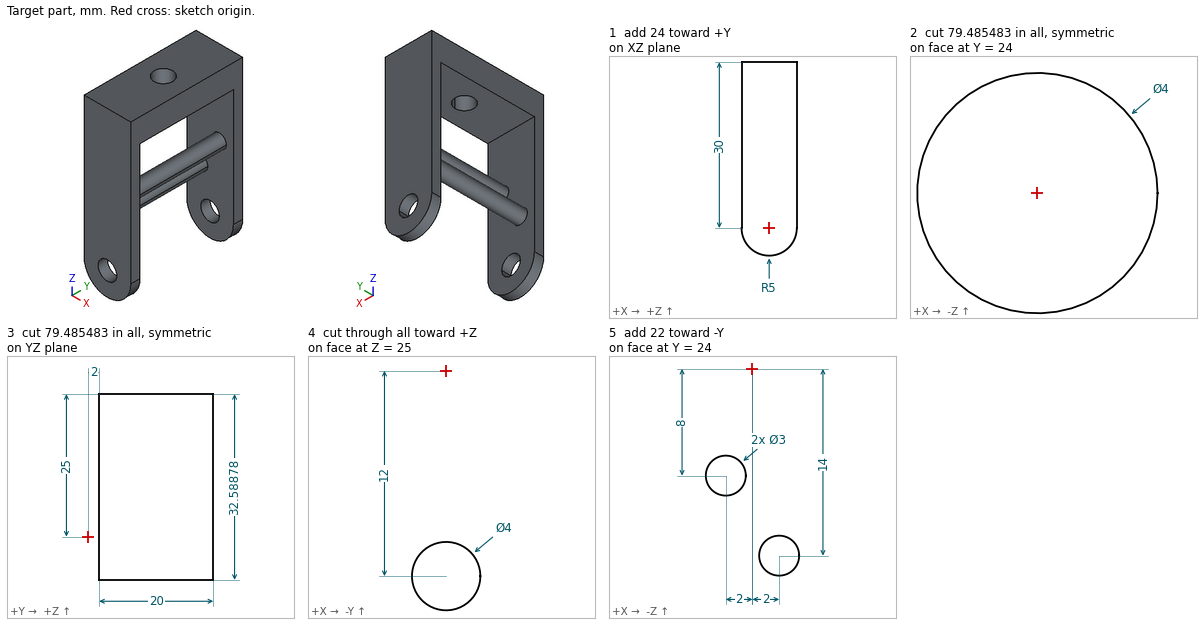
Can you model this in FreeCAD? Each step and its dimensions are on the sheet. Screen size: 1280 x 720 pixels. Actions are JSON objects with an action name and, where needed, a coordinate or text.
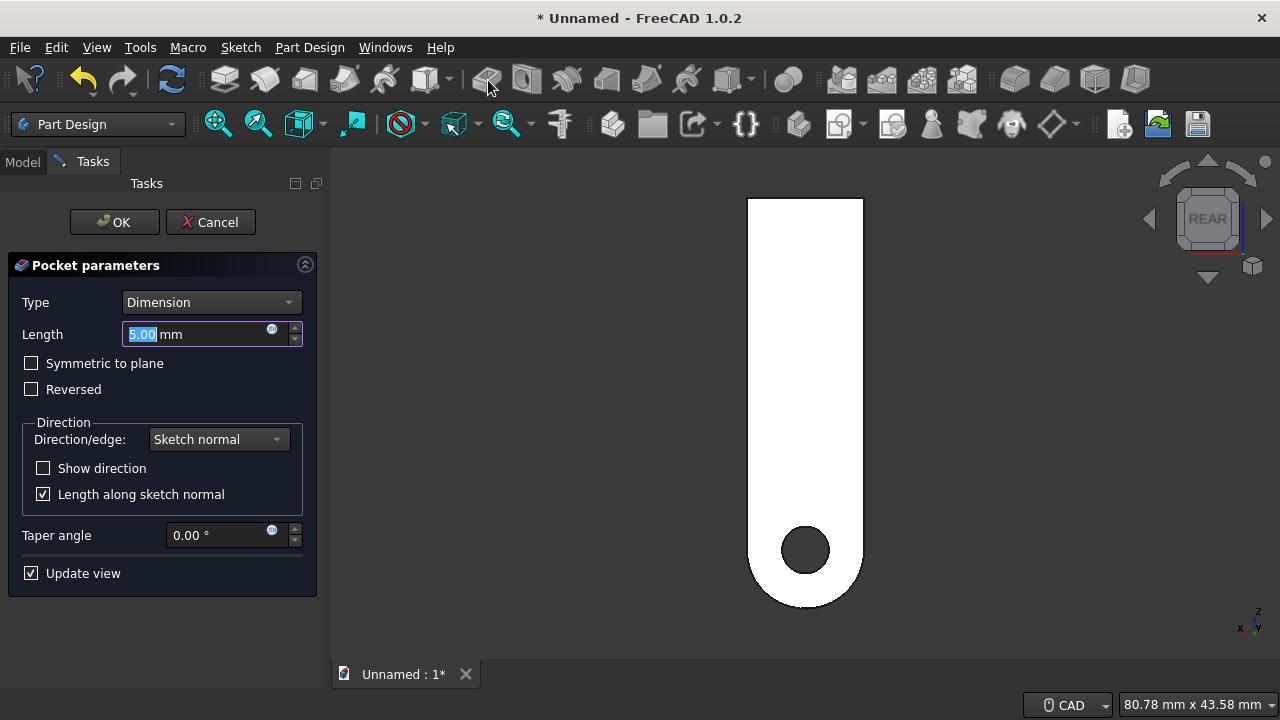
{"action": "type", "text": "79.485483"}
{"action": "key", "text": "Tab"}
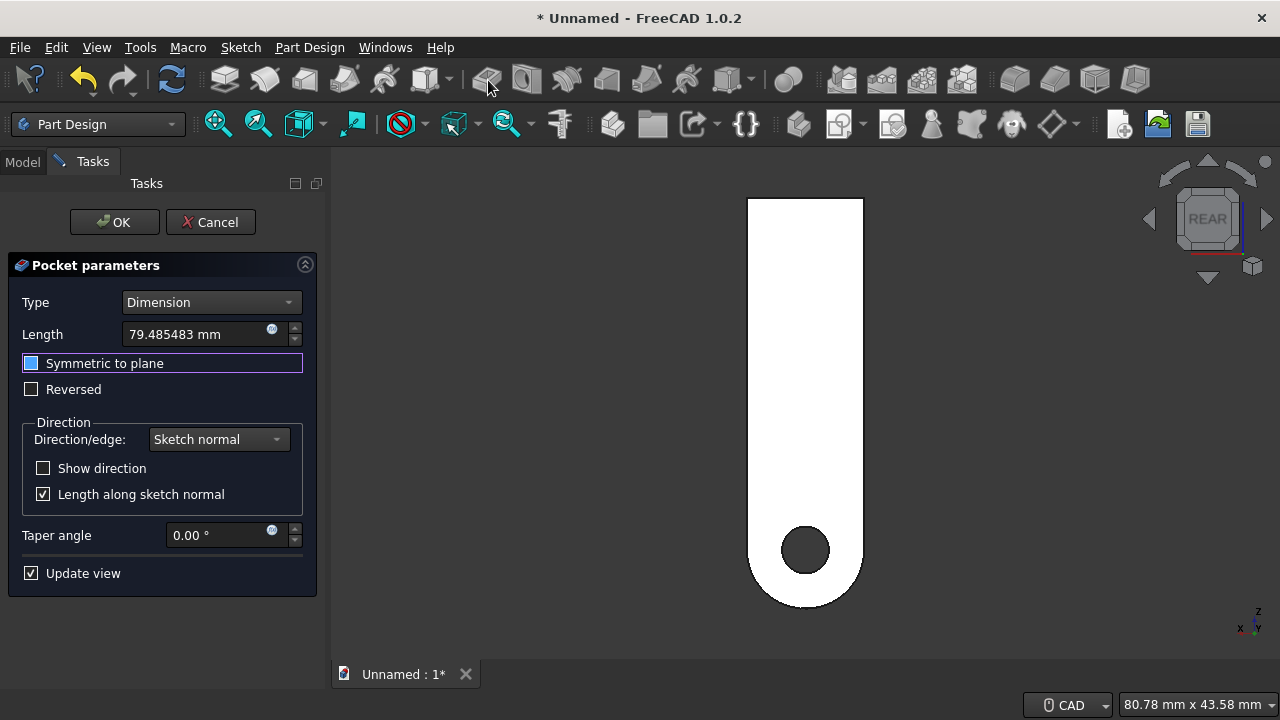
{"action": "left_click", "coordinate": [30, 363]}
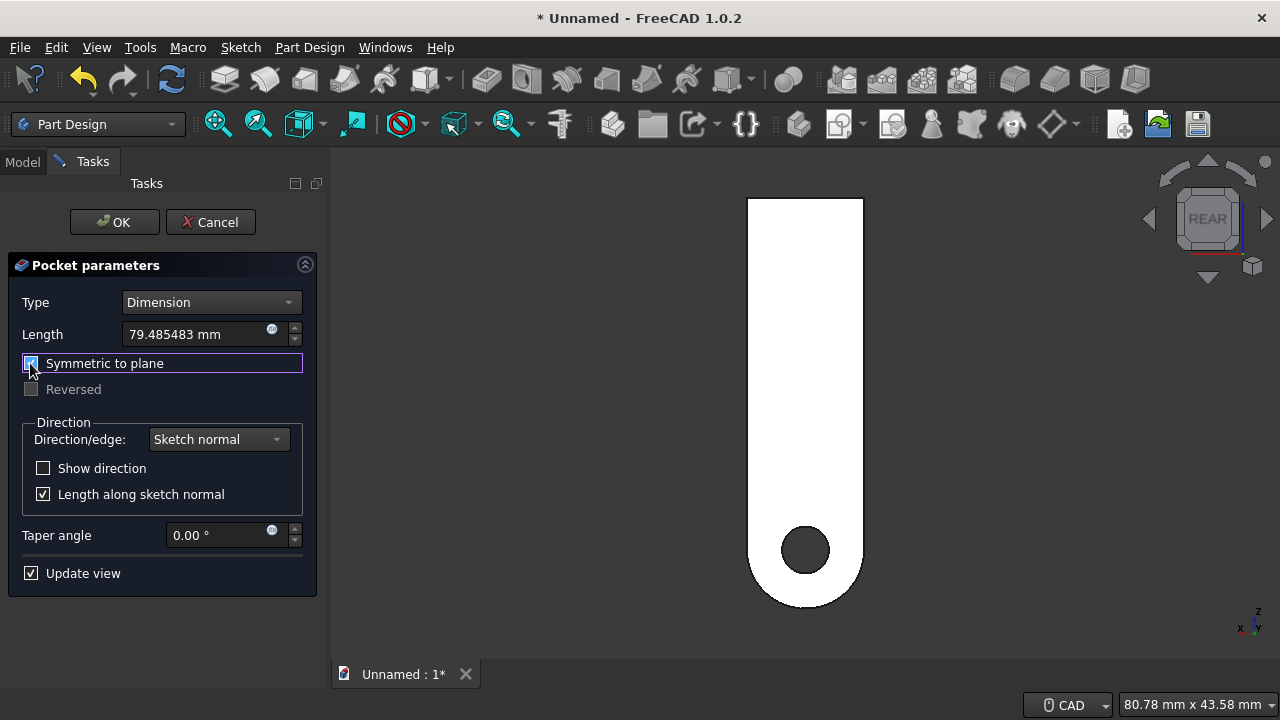
{"action": "left_click", "coordinate": [115, 222]}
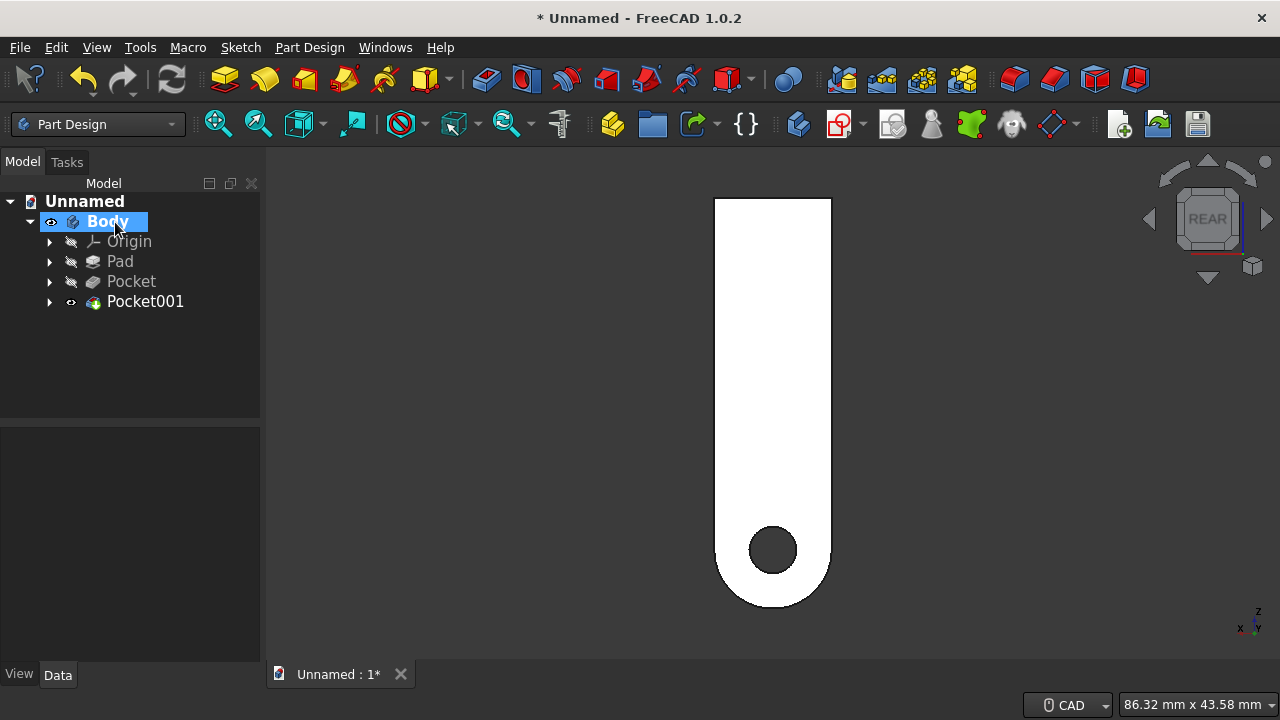
{"action": "key", "text": "5"}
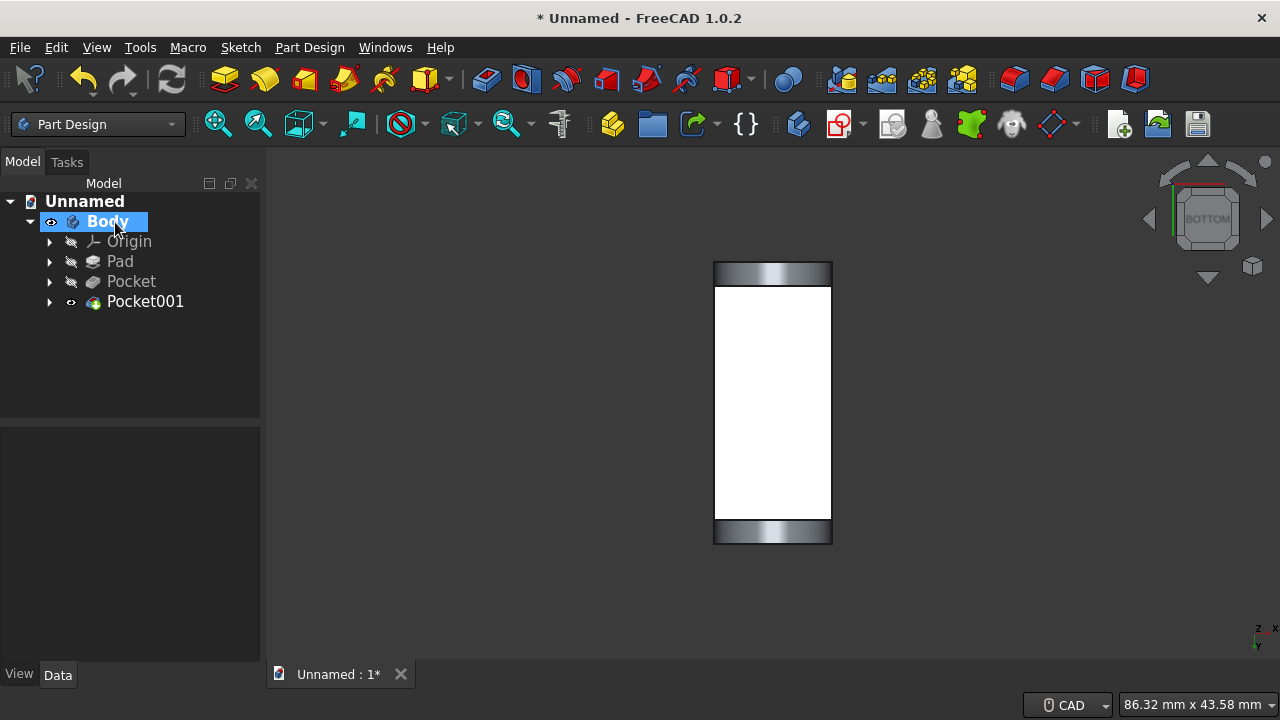
{"action": "left_click", "coordinate": [773, 436]}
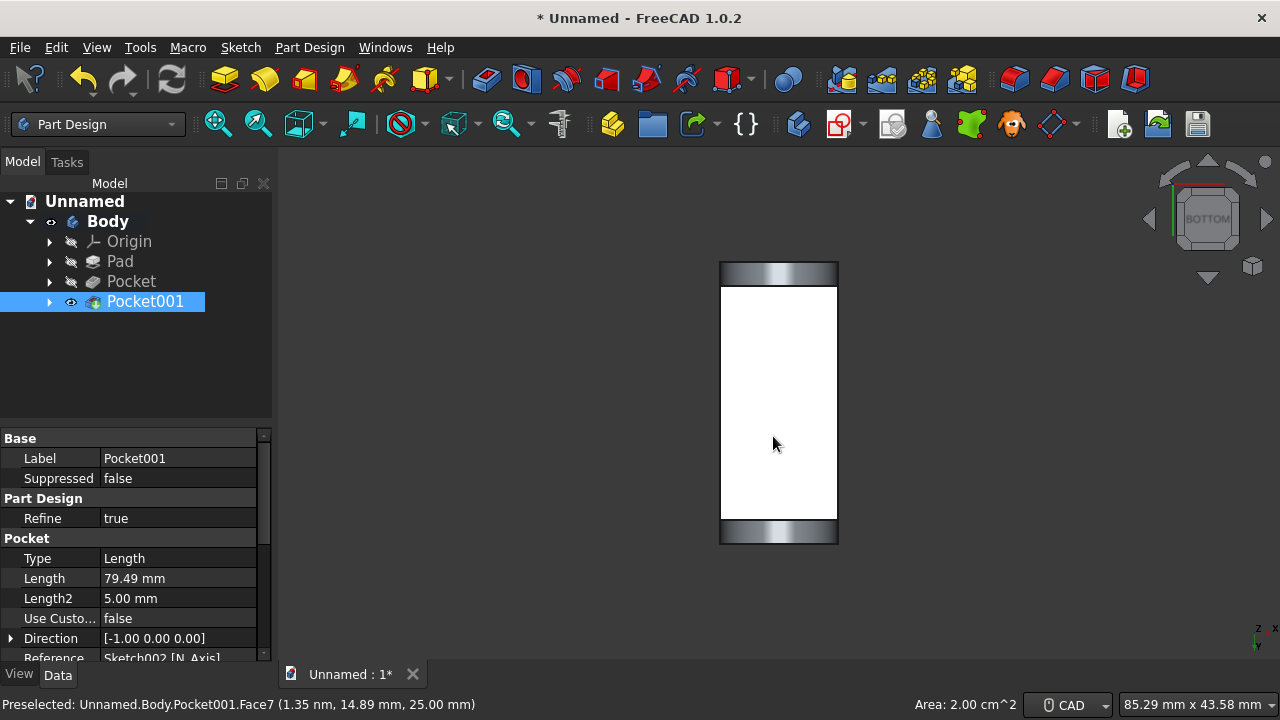
{"action": "left_click", "coordinate": [840, 124]}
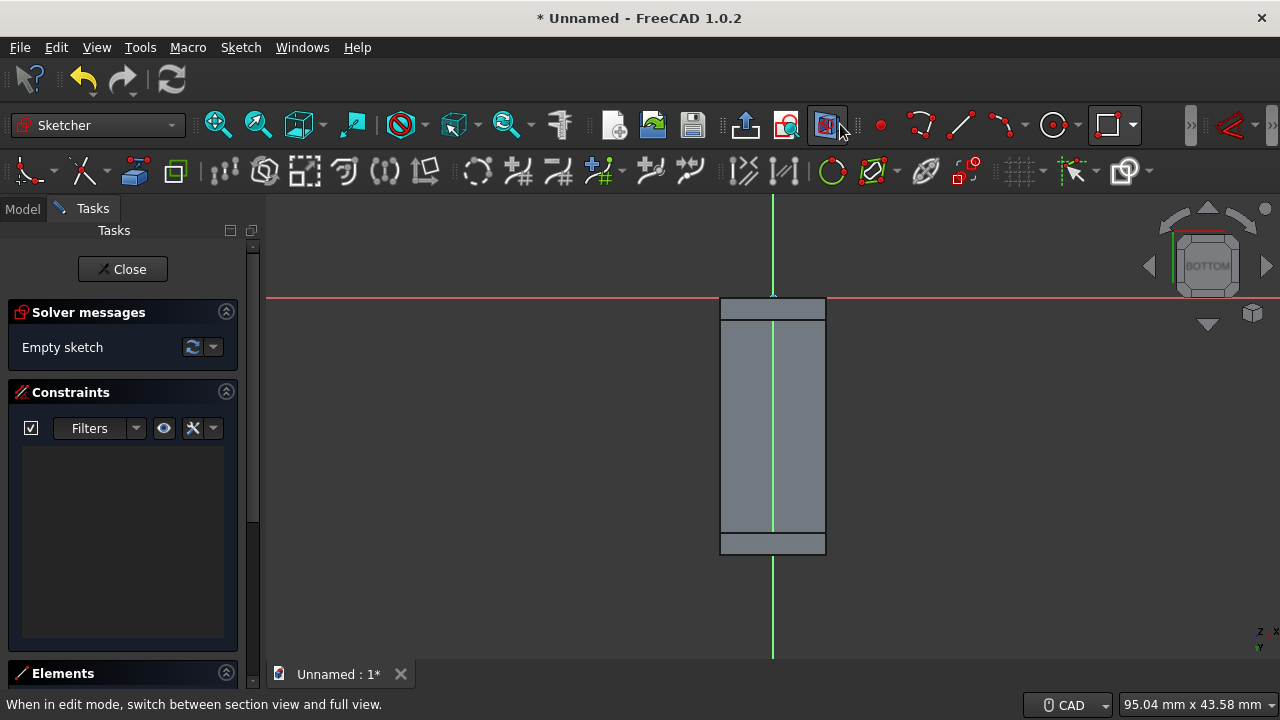
{"action": "scroll", "coordinate": [784, 427], "scroll_direction": "up", "scroll_amount": 10}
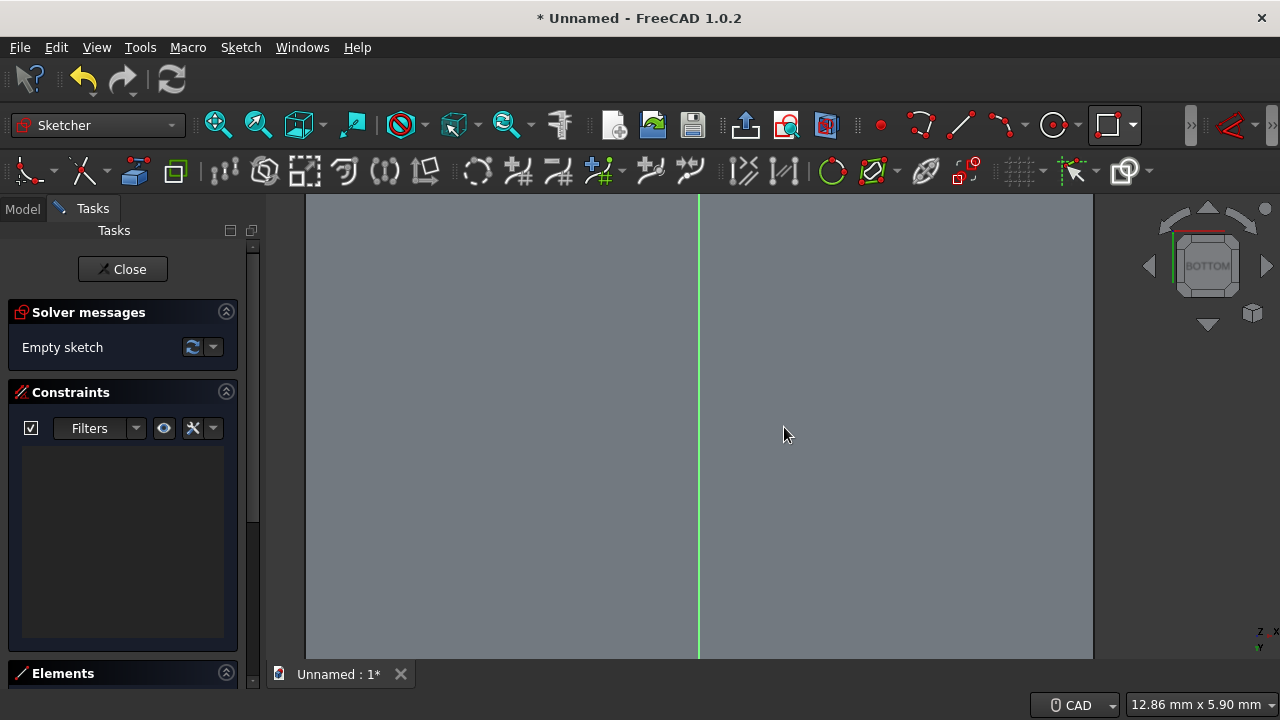
{"action": "left_click", "coordinate": [1054, 126]}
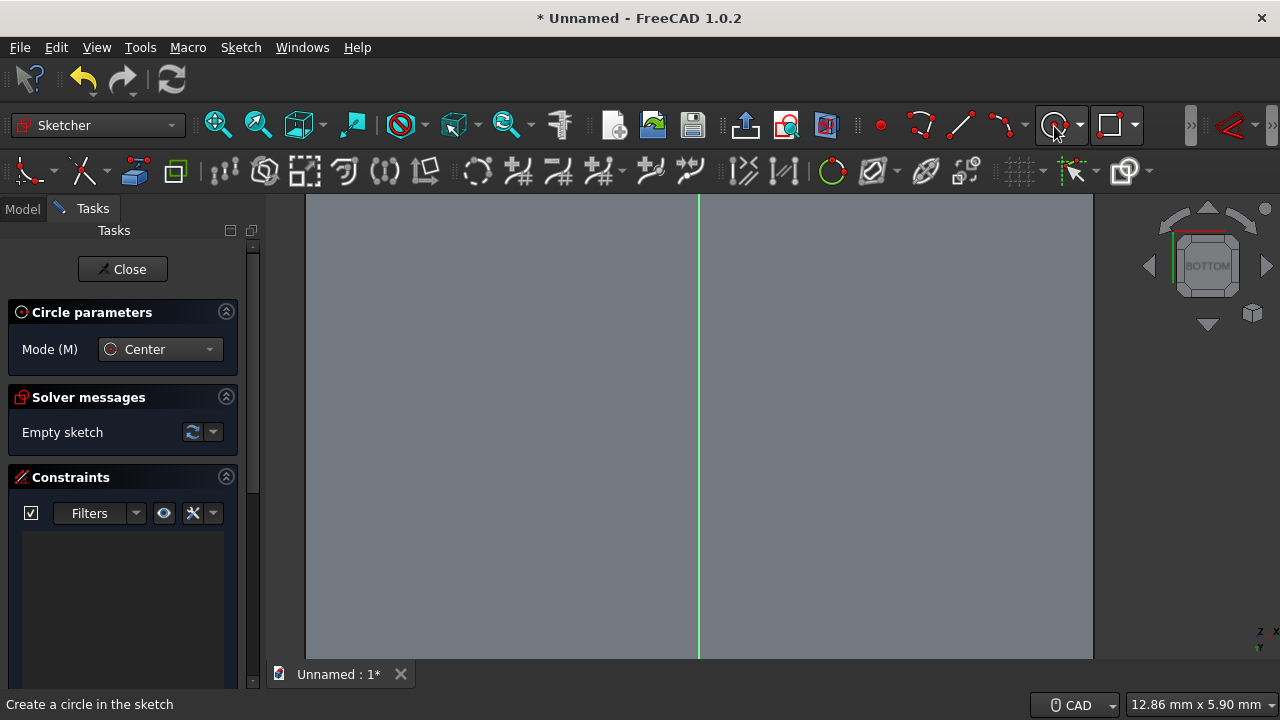
{"action": "left_click", "coordinate": [699, 420]}
{"action": "mouse_move", "coordinate": [811, 309]}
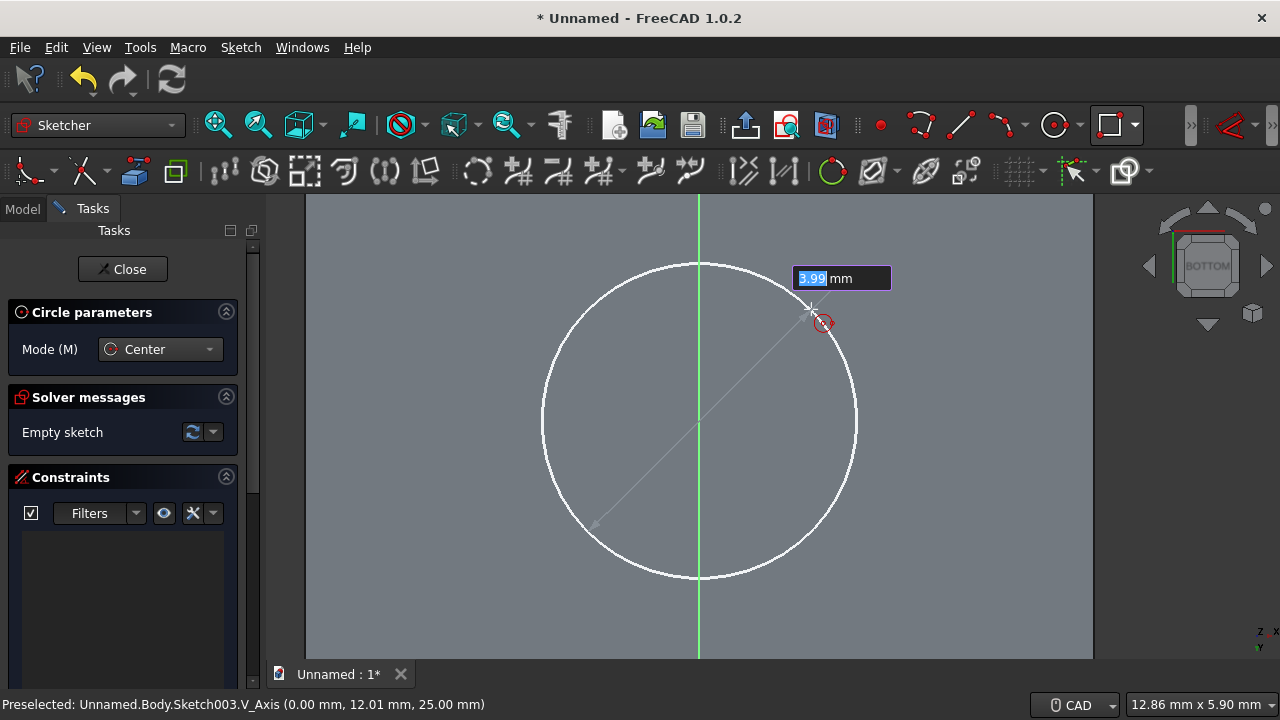
{"action": "type", "text": "4"}
{"action": "key", "text": "Return"}
{"action": "key", "text": "Escape"}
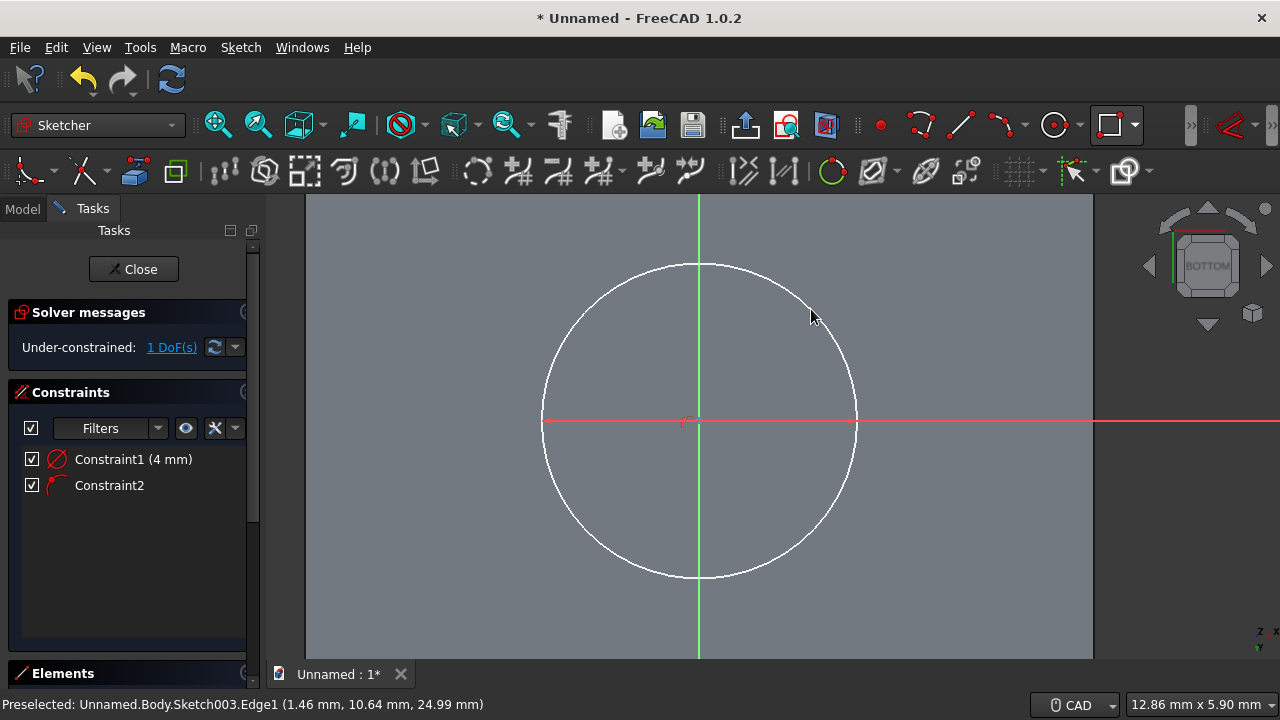
{"action": "left_click", "coordinate": [1230, 126]}